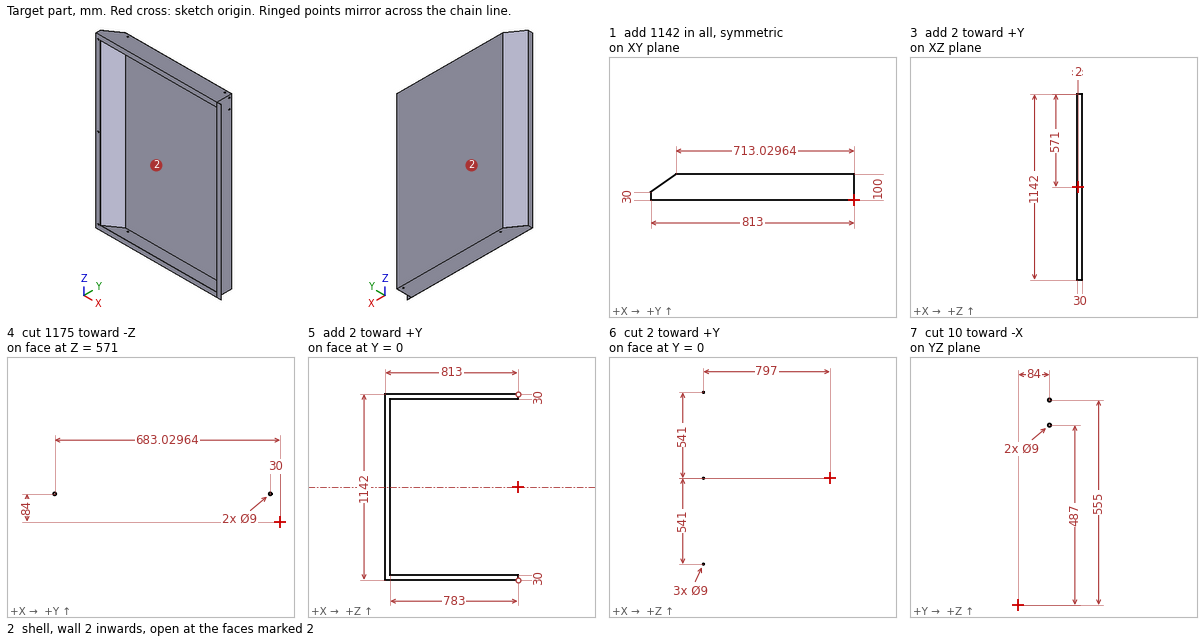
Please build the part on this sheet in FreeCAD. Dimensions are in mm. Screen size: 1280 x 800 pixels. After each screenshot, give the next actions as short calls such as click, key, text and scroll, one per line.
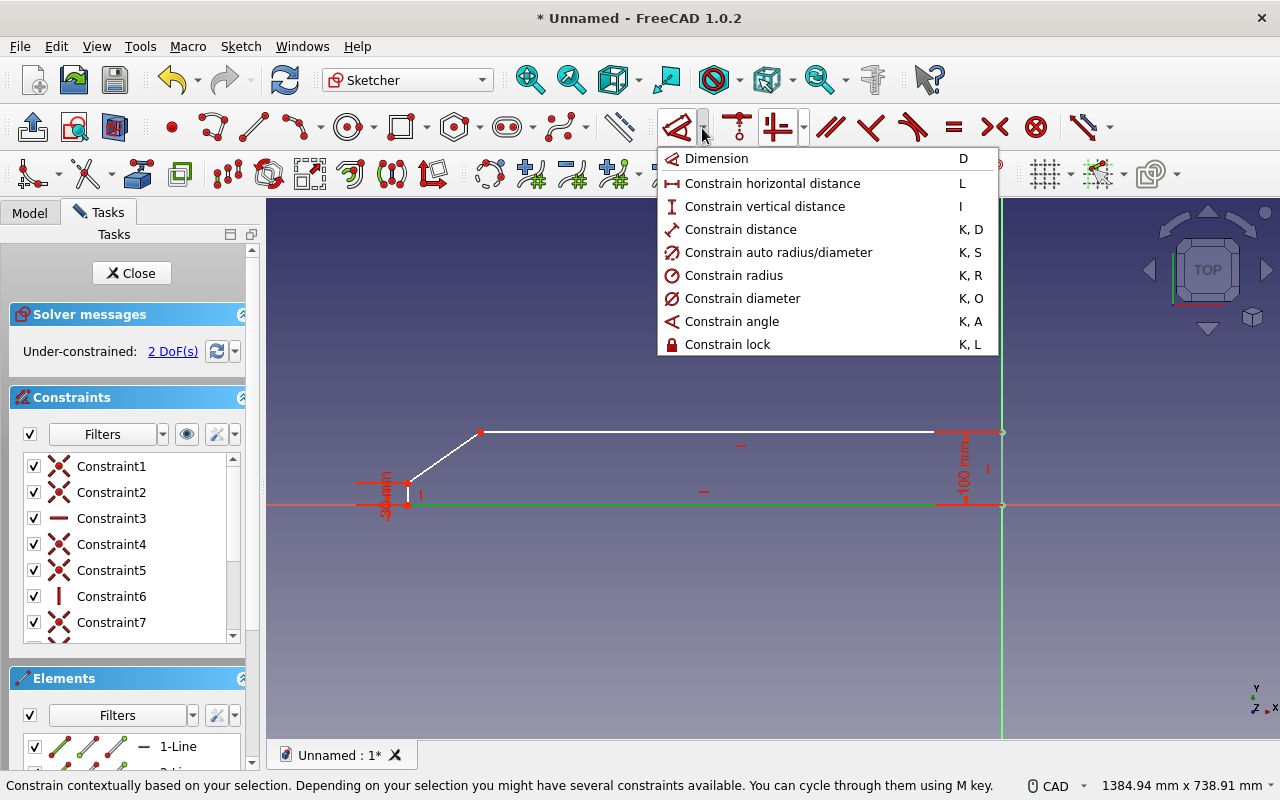
click(828, 184)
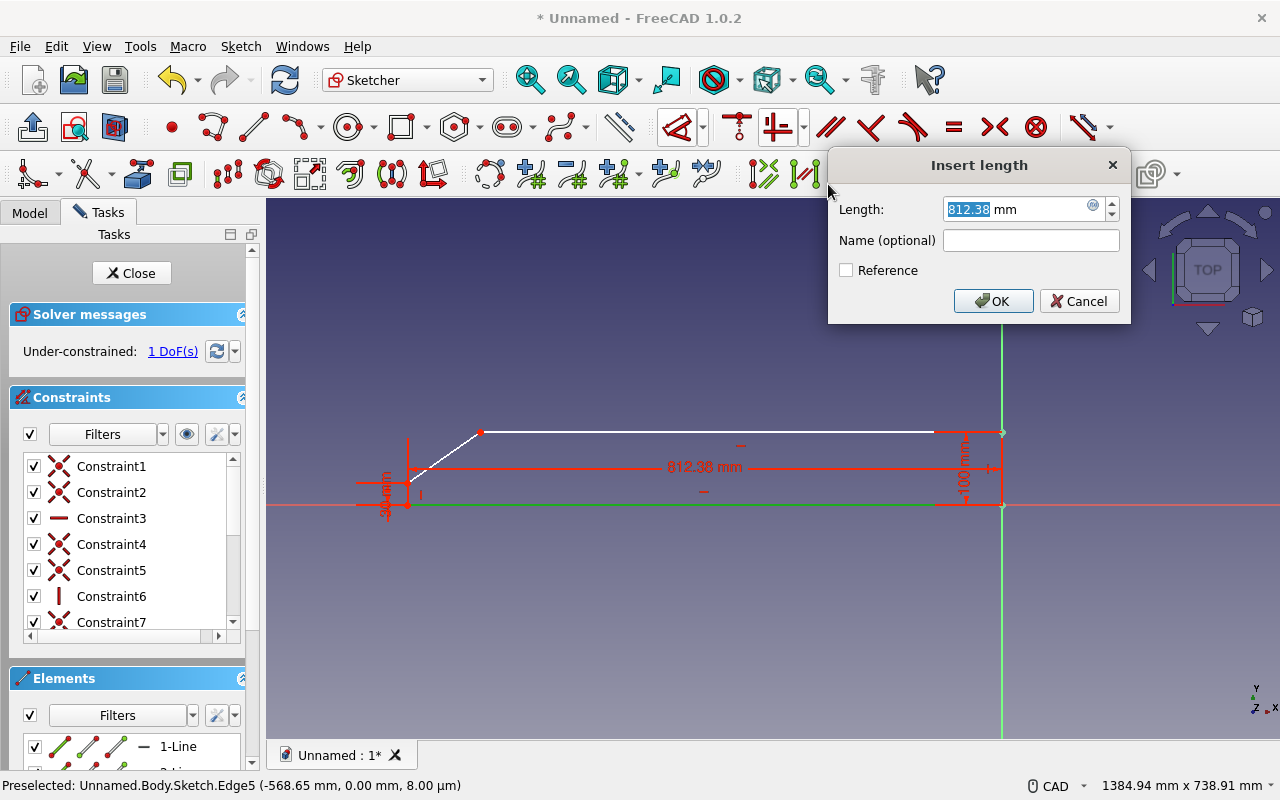
text(813)
key(Return)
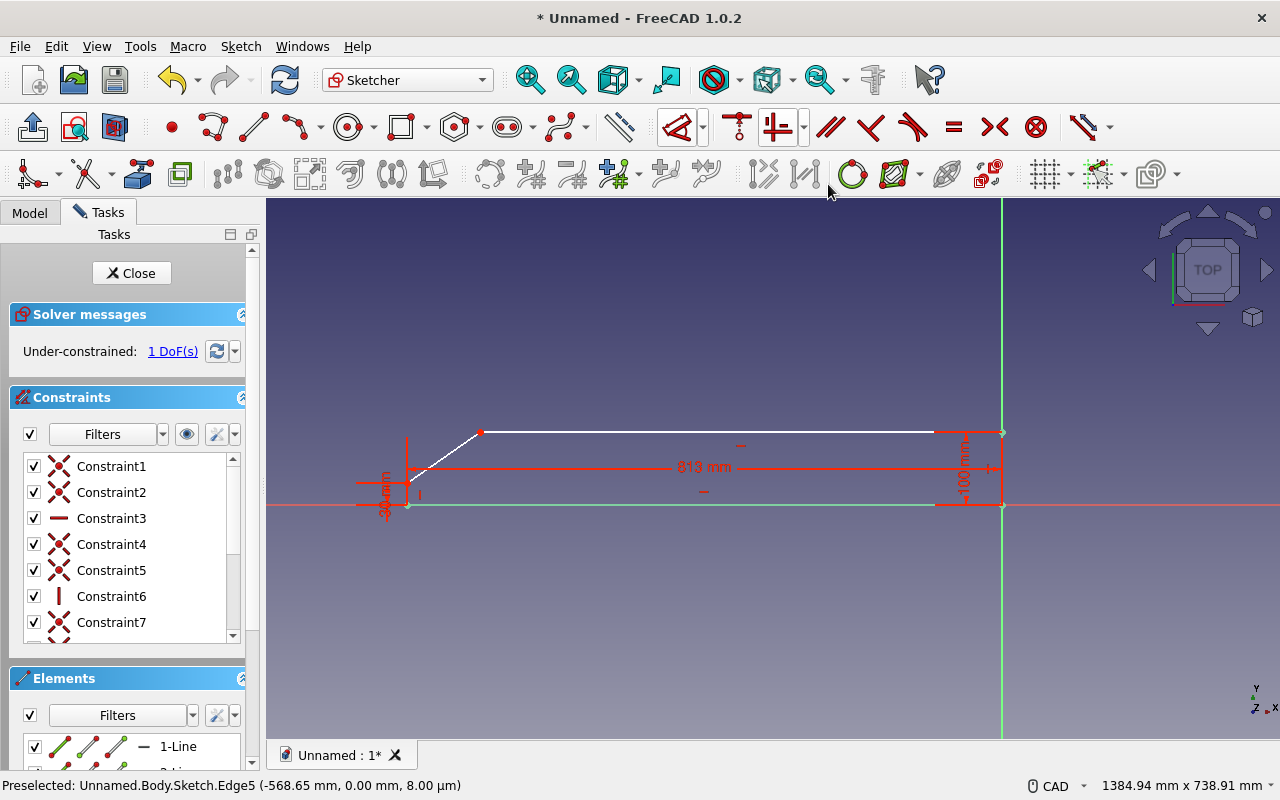
click(846, 432)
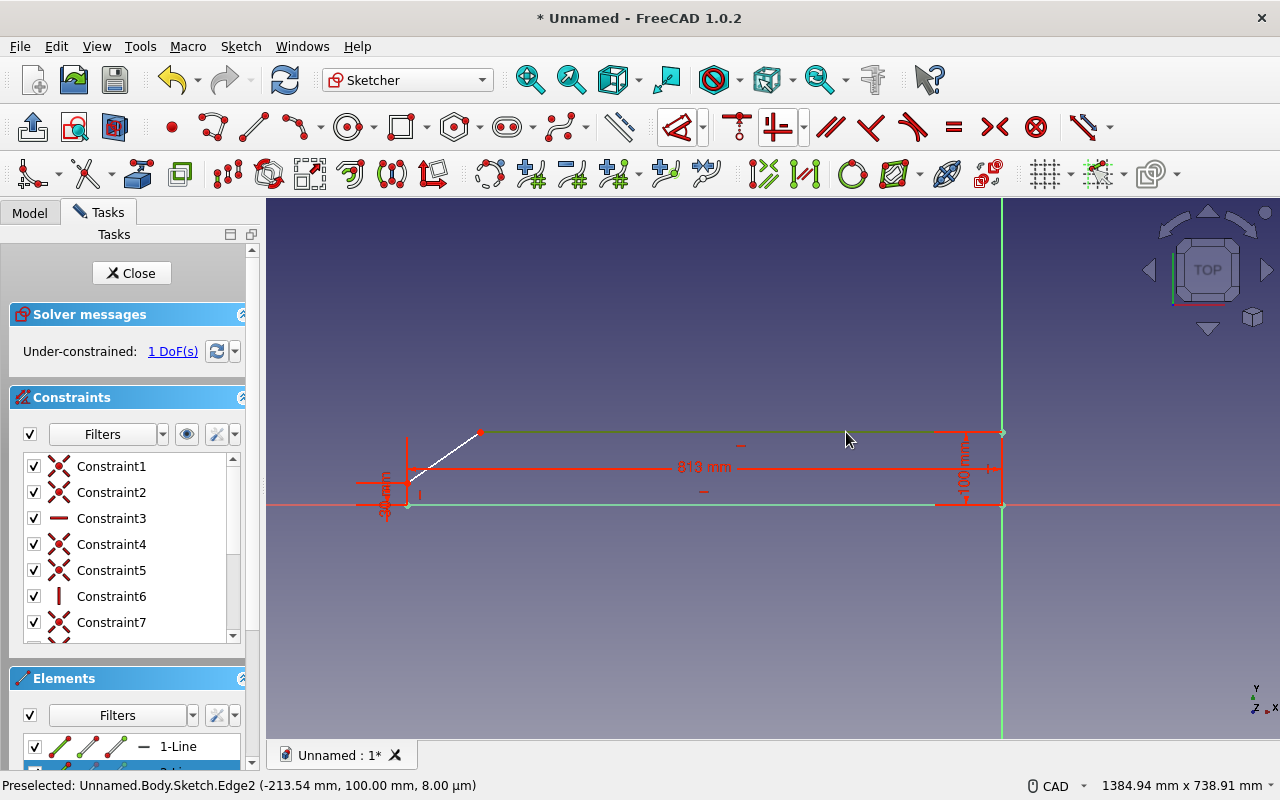
key(l)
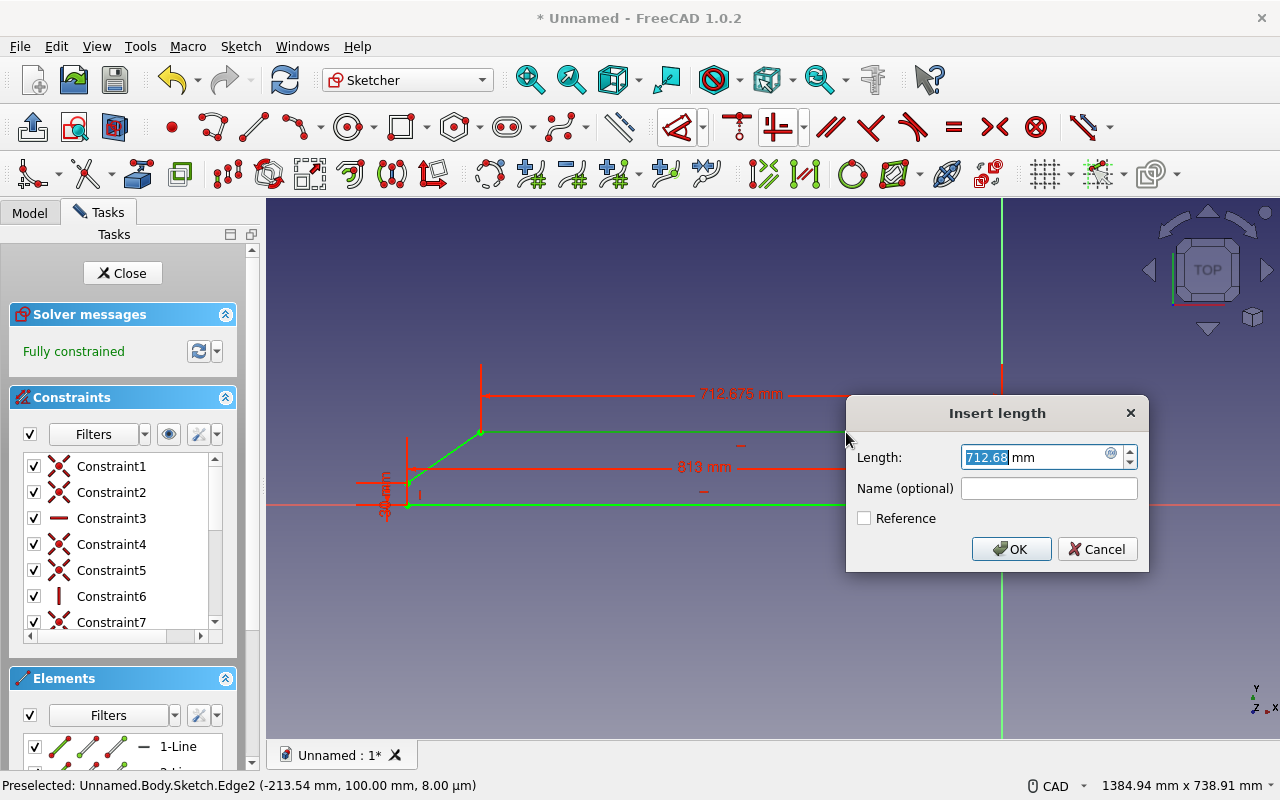
text(713.02964)
key(Return)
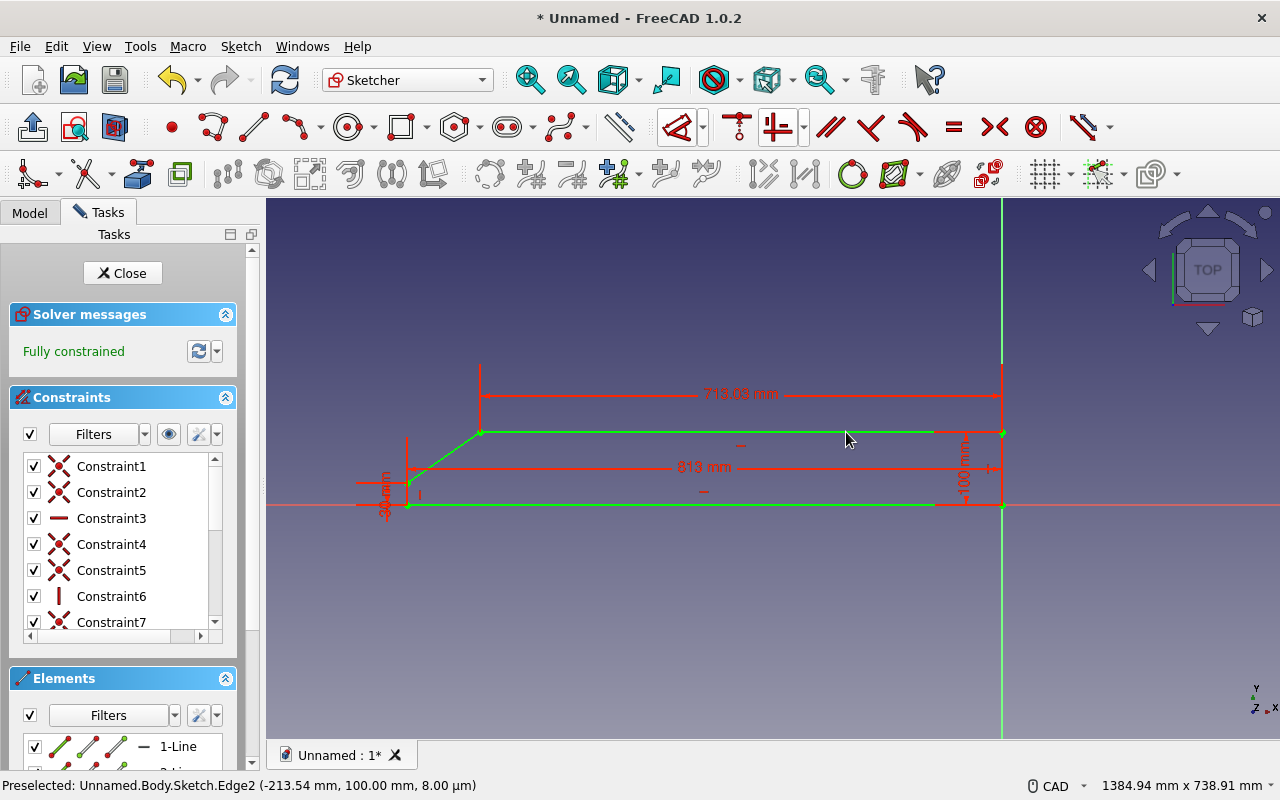
click(123, 273)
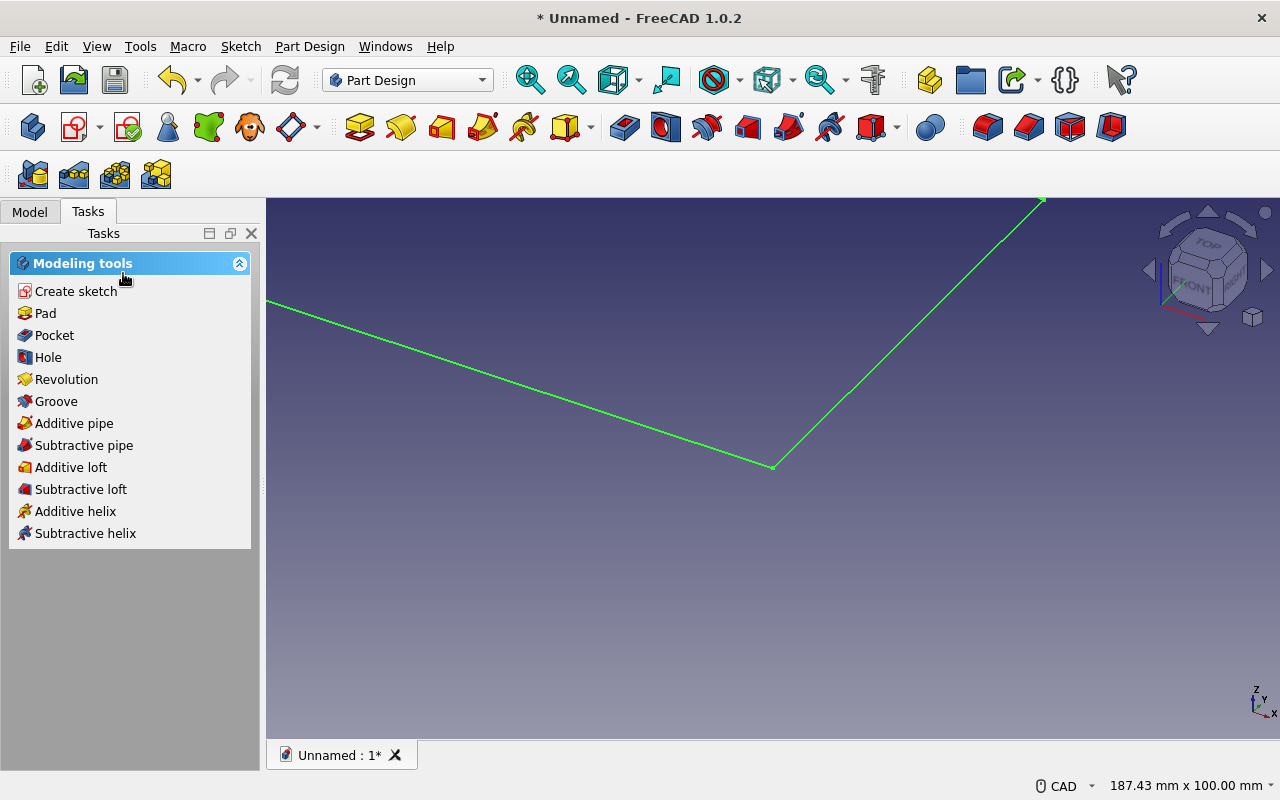
click(360, 128)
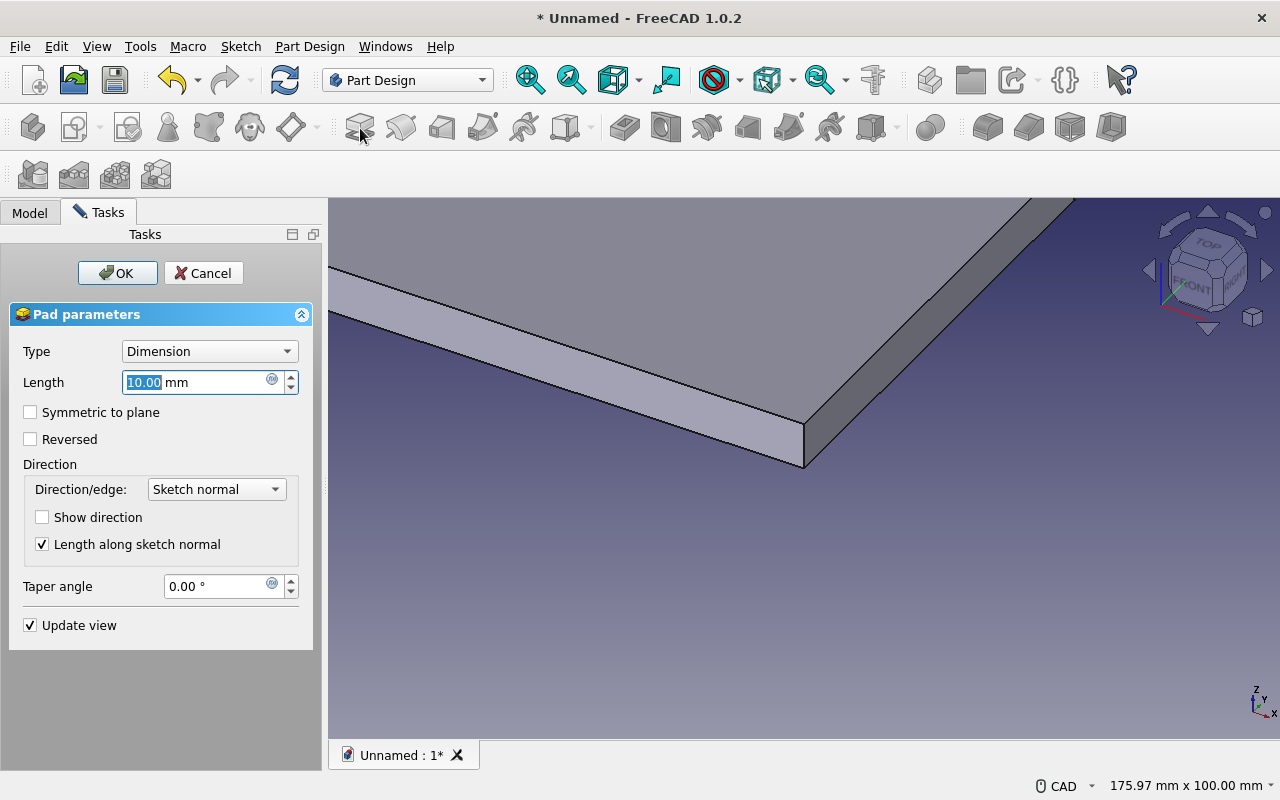
text(1142)
key(Tab)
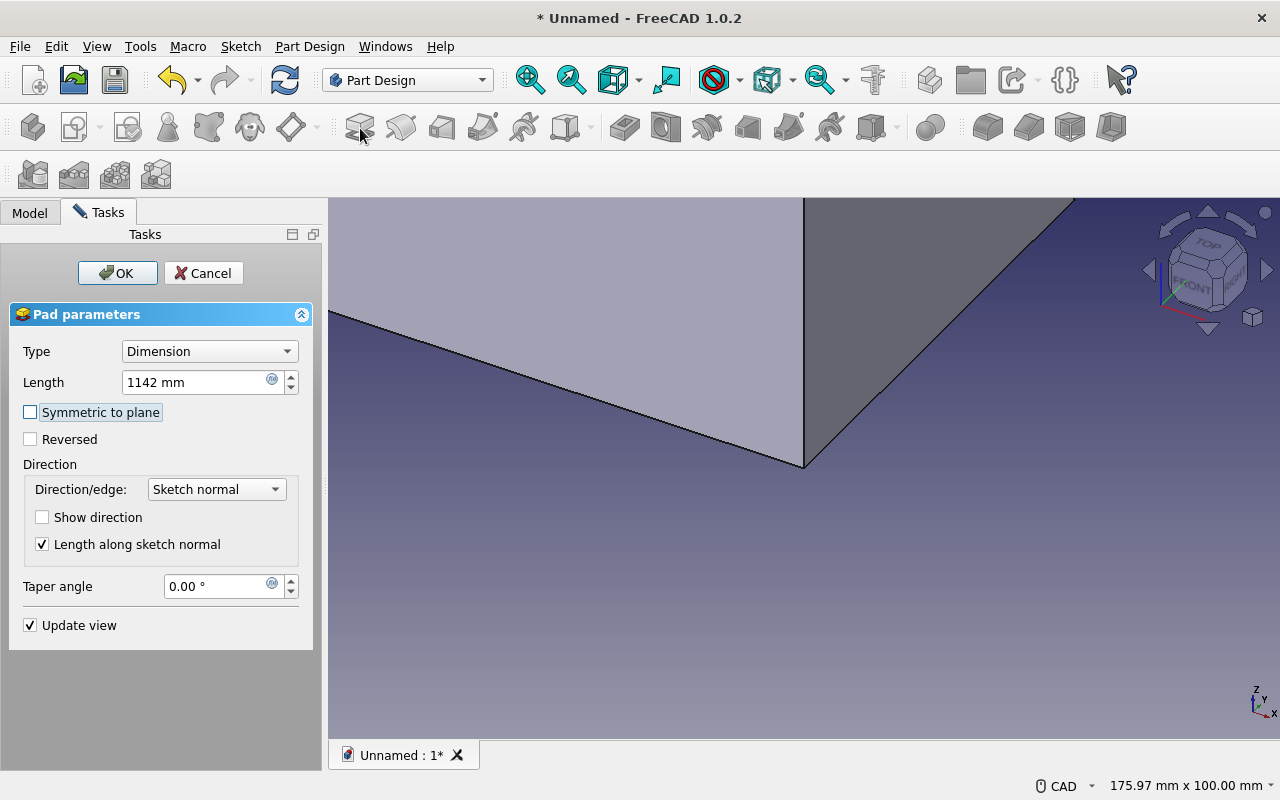
click(31, 412)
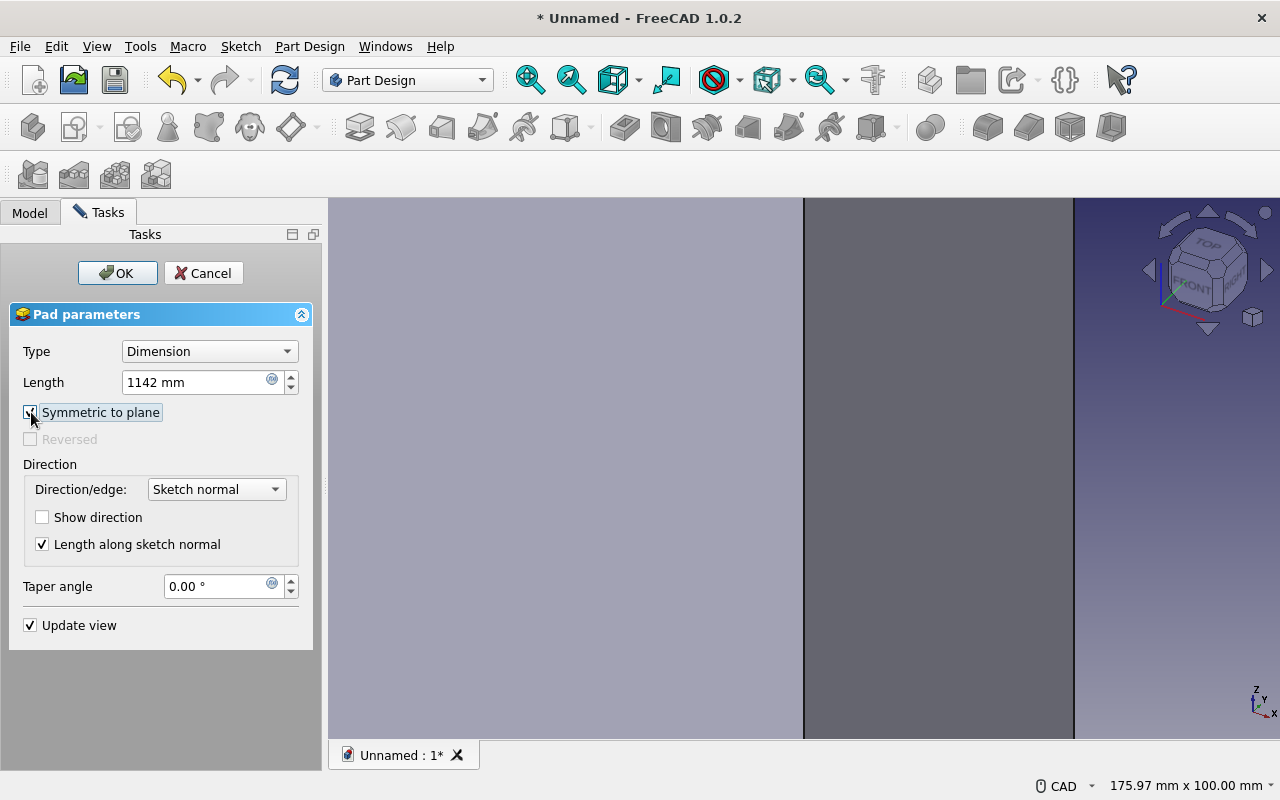
click(118, 273)